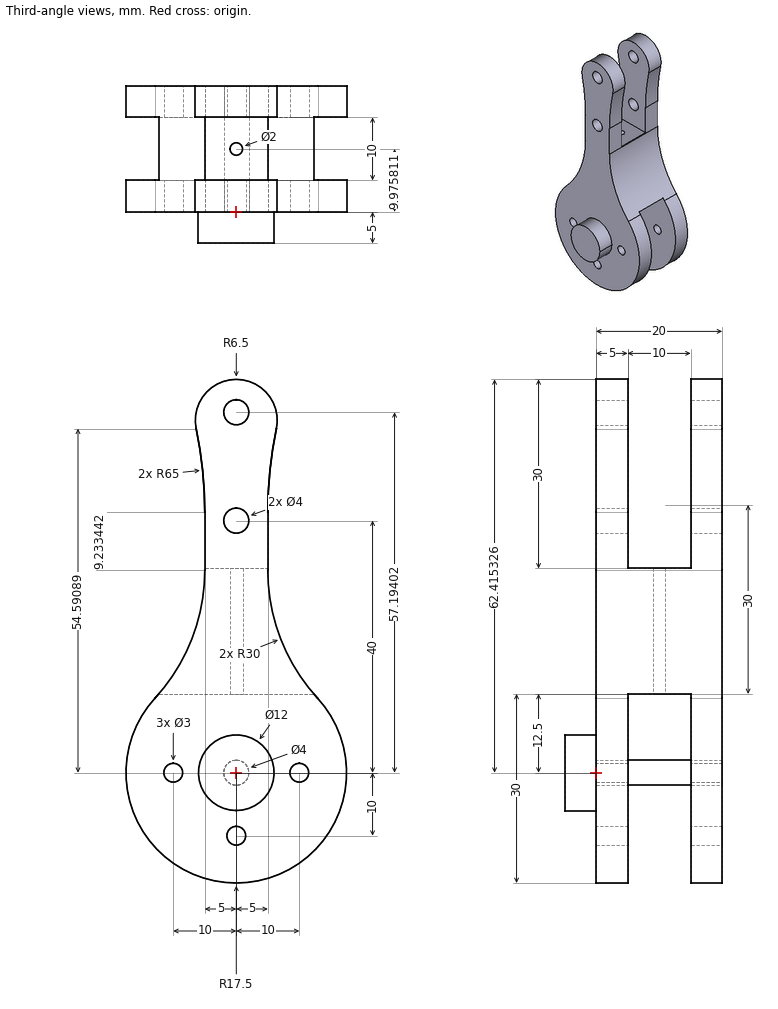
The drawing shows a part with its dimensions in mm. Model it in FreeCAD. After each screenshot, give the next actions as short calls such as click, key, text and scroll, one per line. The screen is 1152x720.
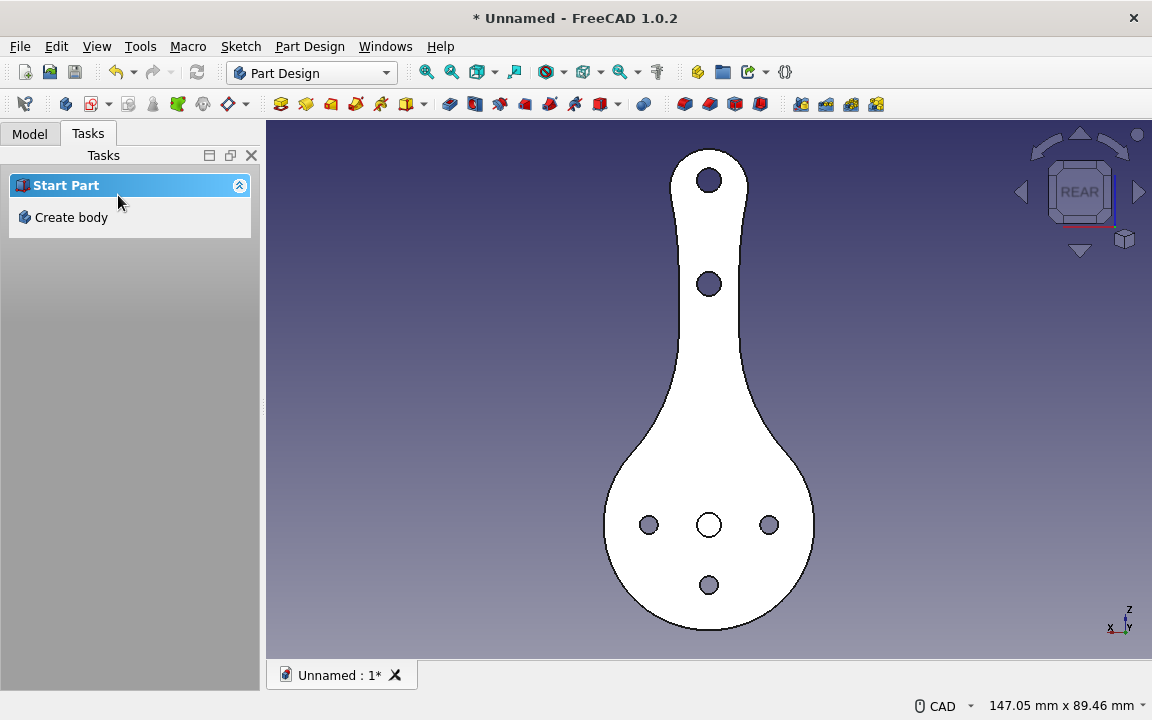
key(5)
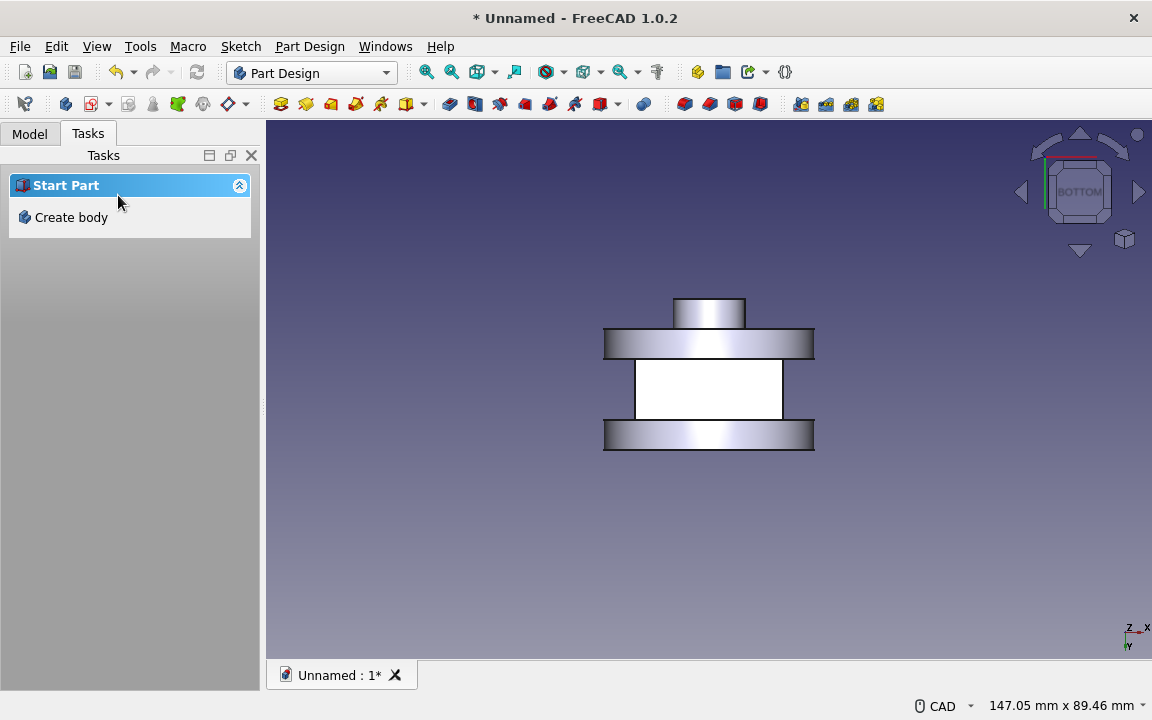
click(427, 72)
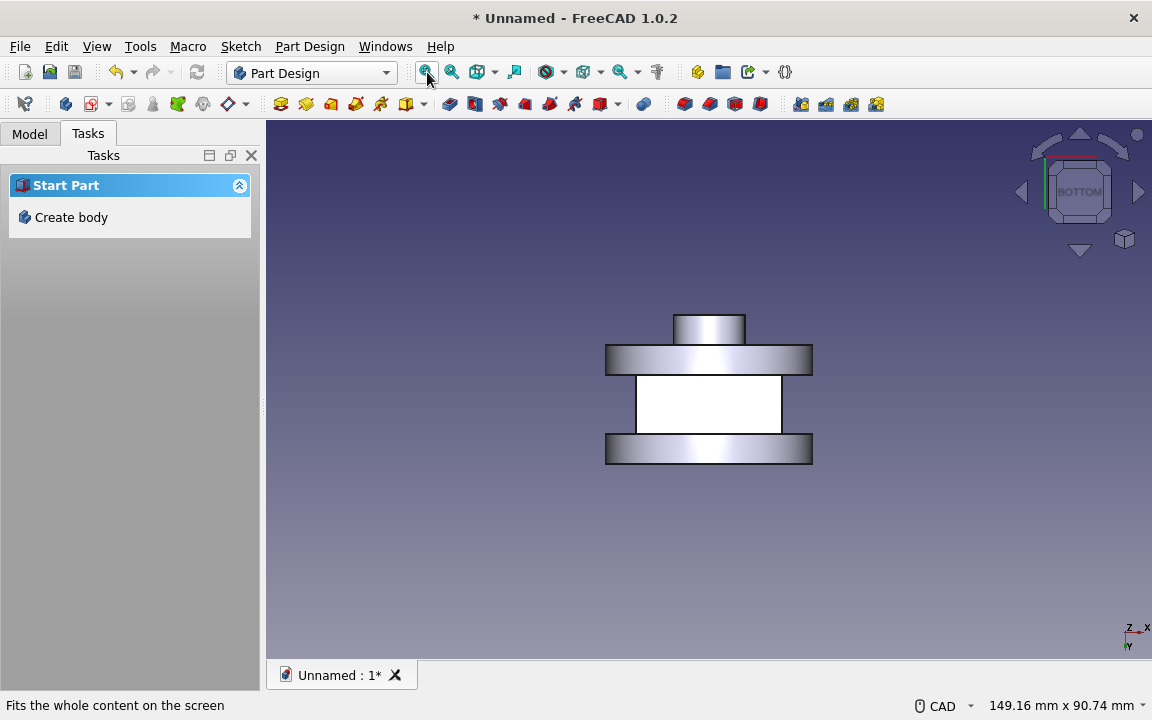
click(751, 403)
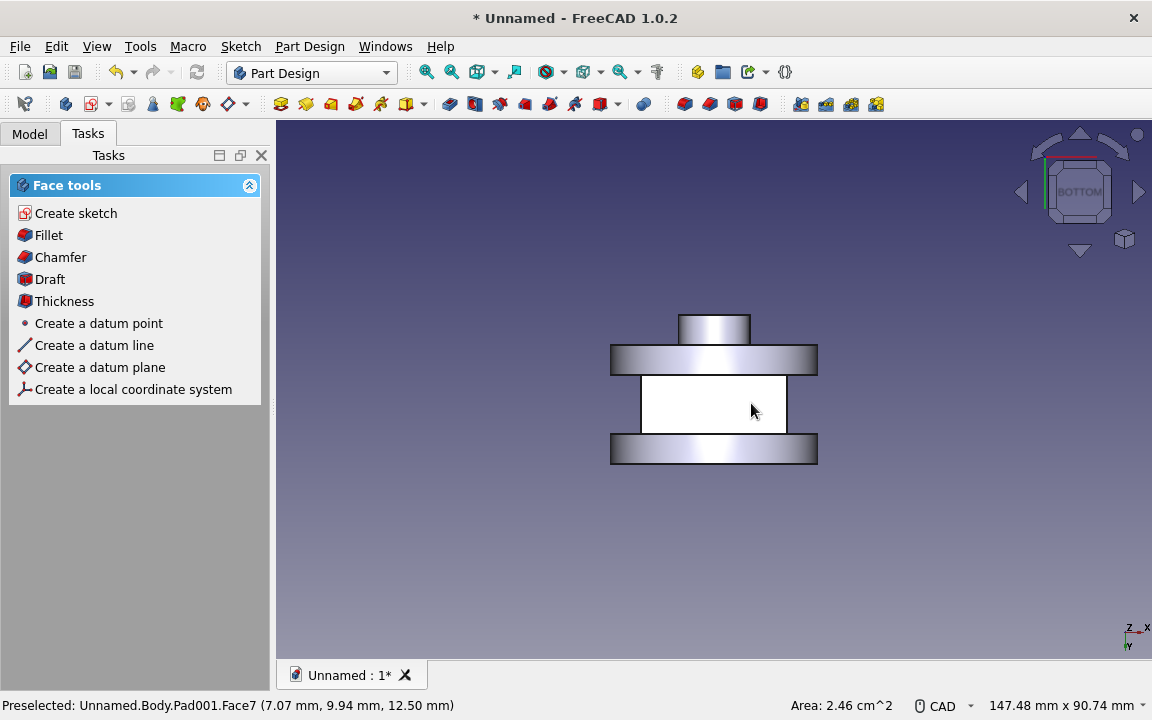
click(90, 104)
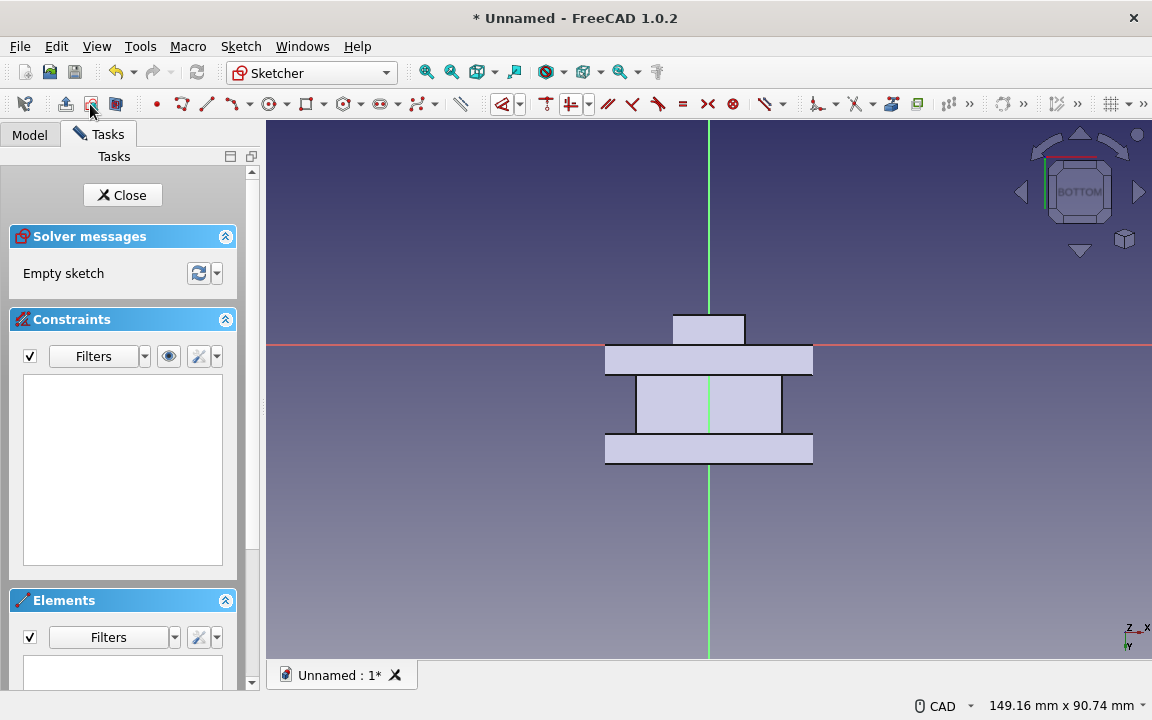
scroll(713, 405, up, 15)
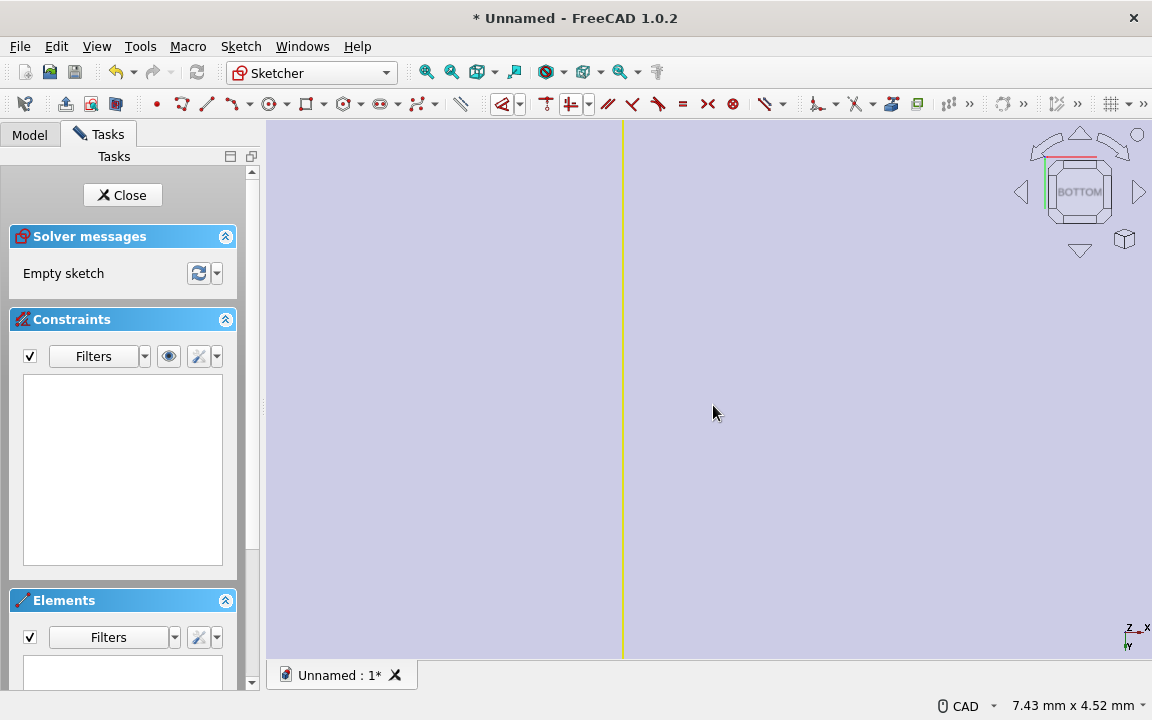
scroll(587, 357, up, 2)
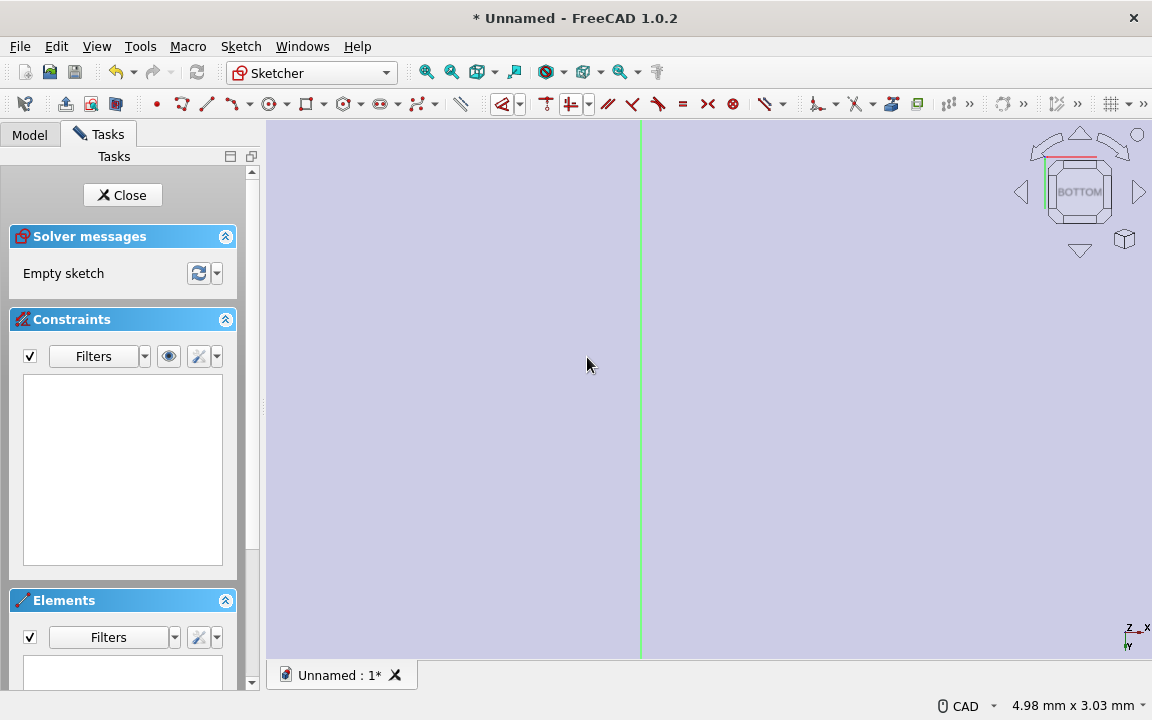
click(268, 104)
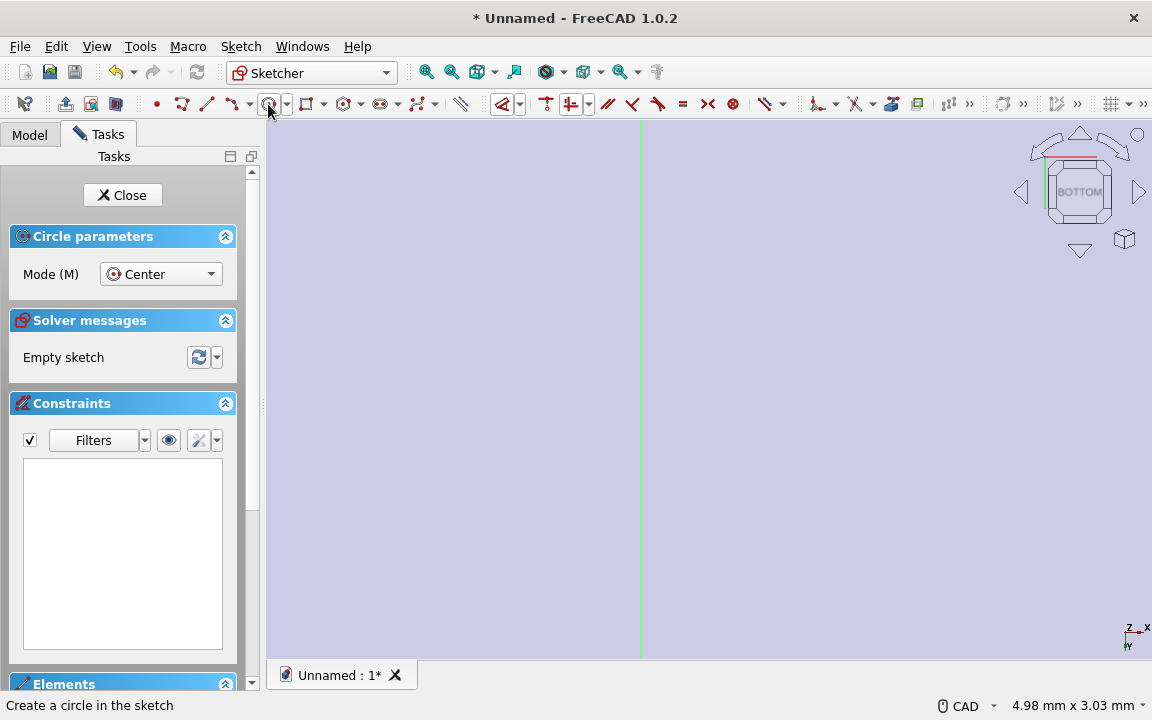
click(641, 390)
click(766, 264)
key(Escape)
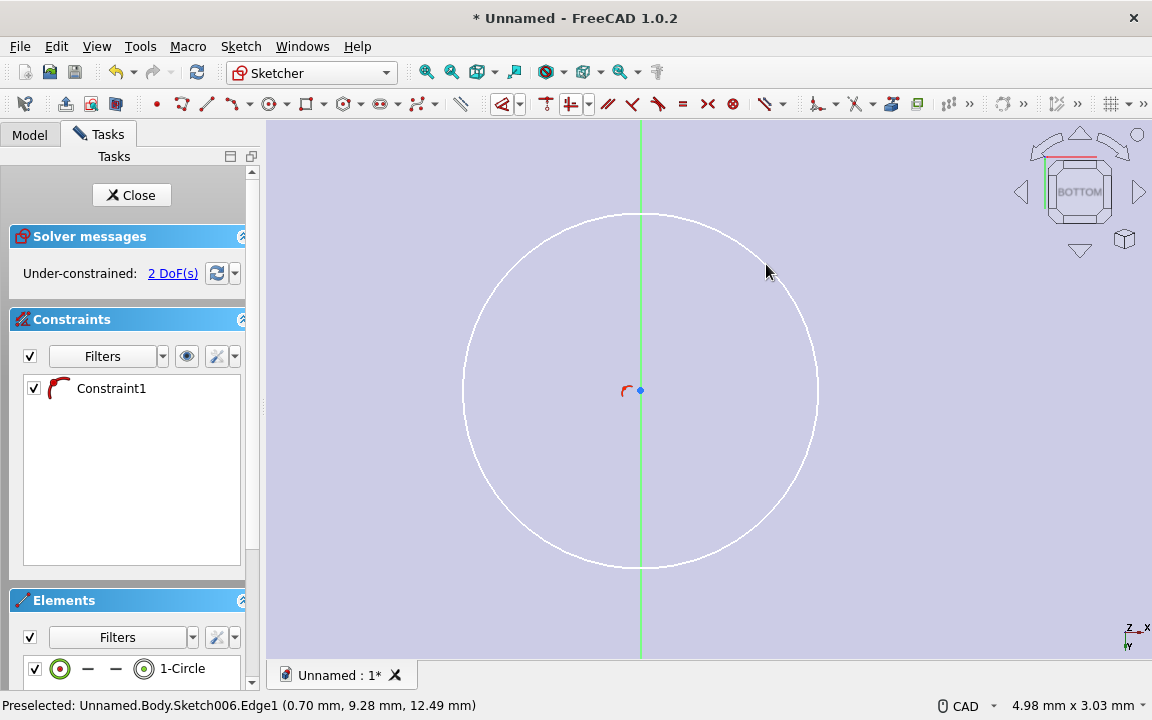
click(766, 265)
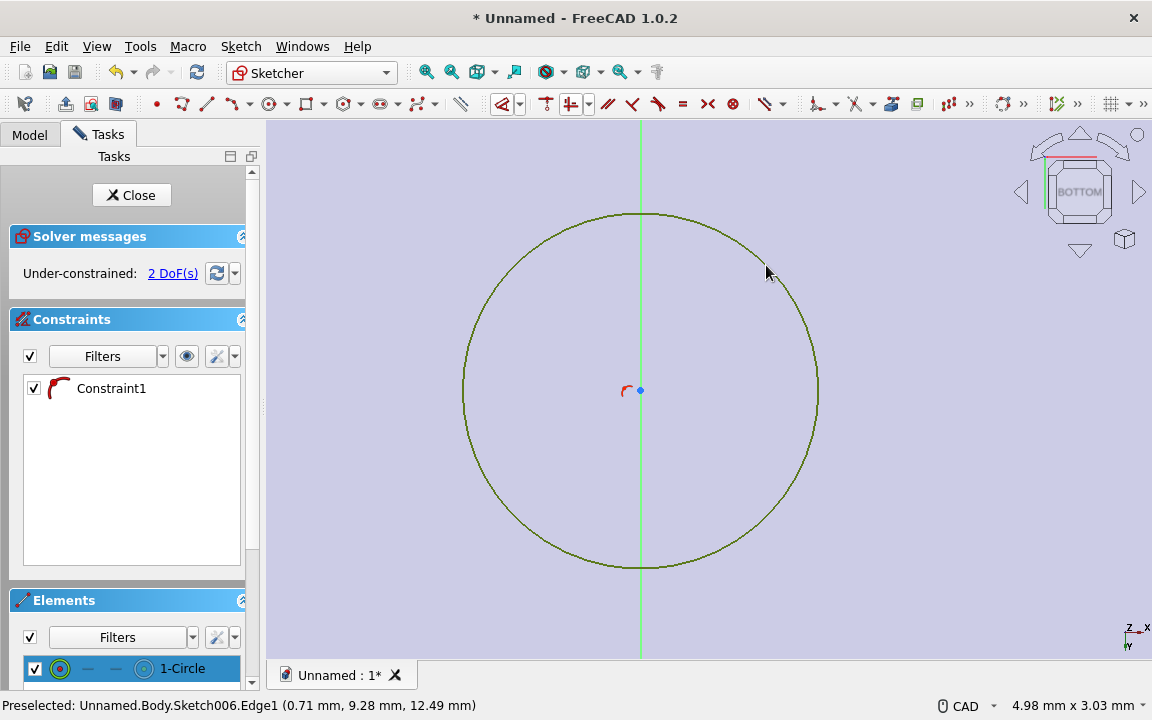
key(k)
key(o)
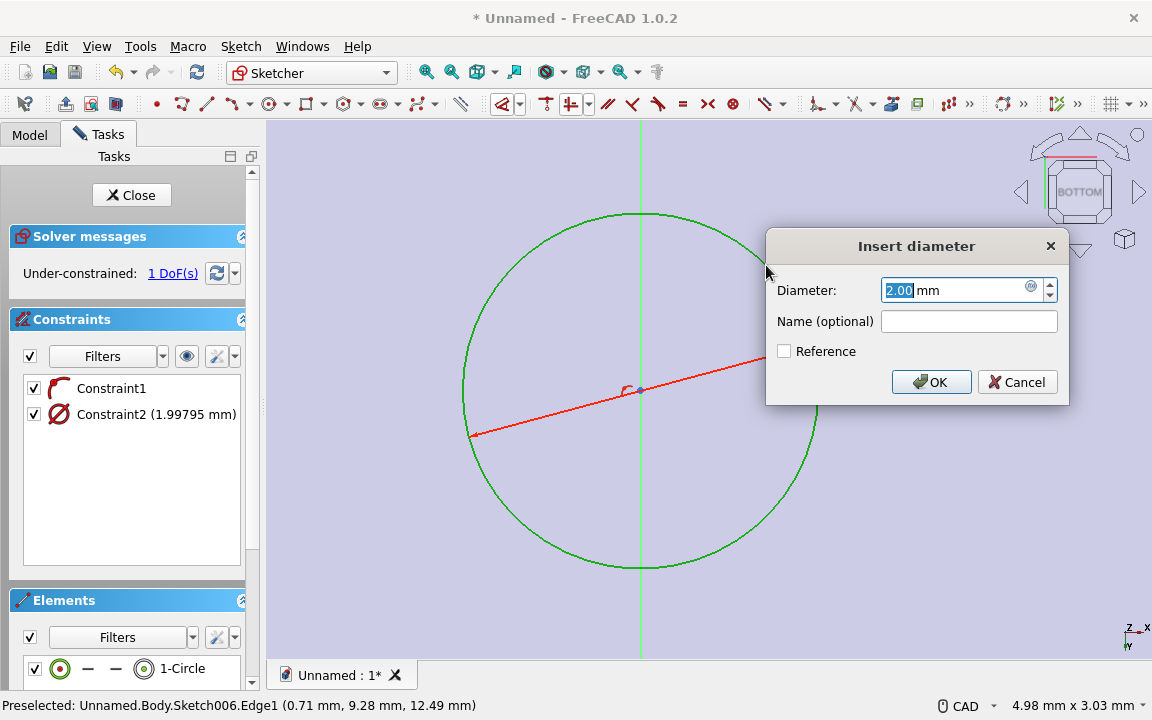
text(2)
key(Return)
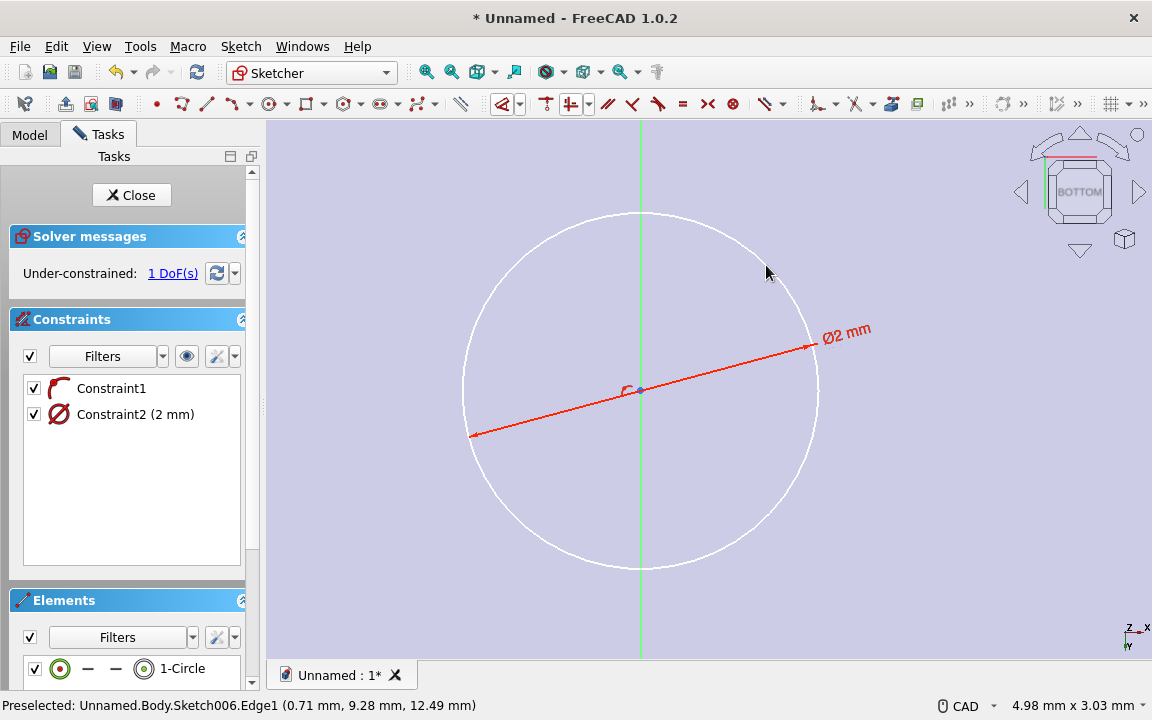
click(641, 391)